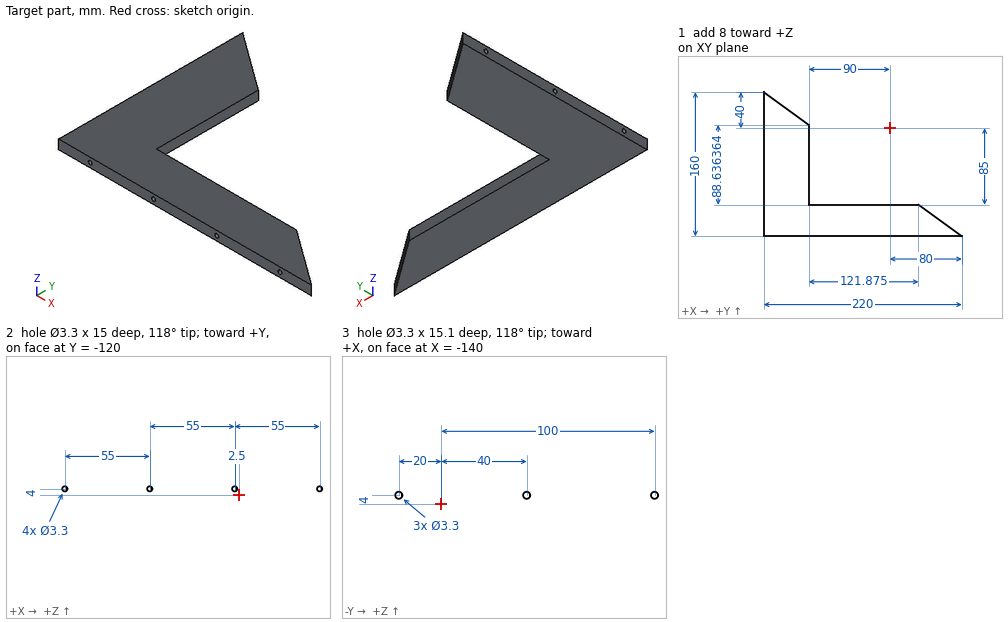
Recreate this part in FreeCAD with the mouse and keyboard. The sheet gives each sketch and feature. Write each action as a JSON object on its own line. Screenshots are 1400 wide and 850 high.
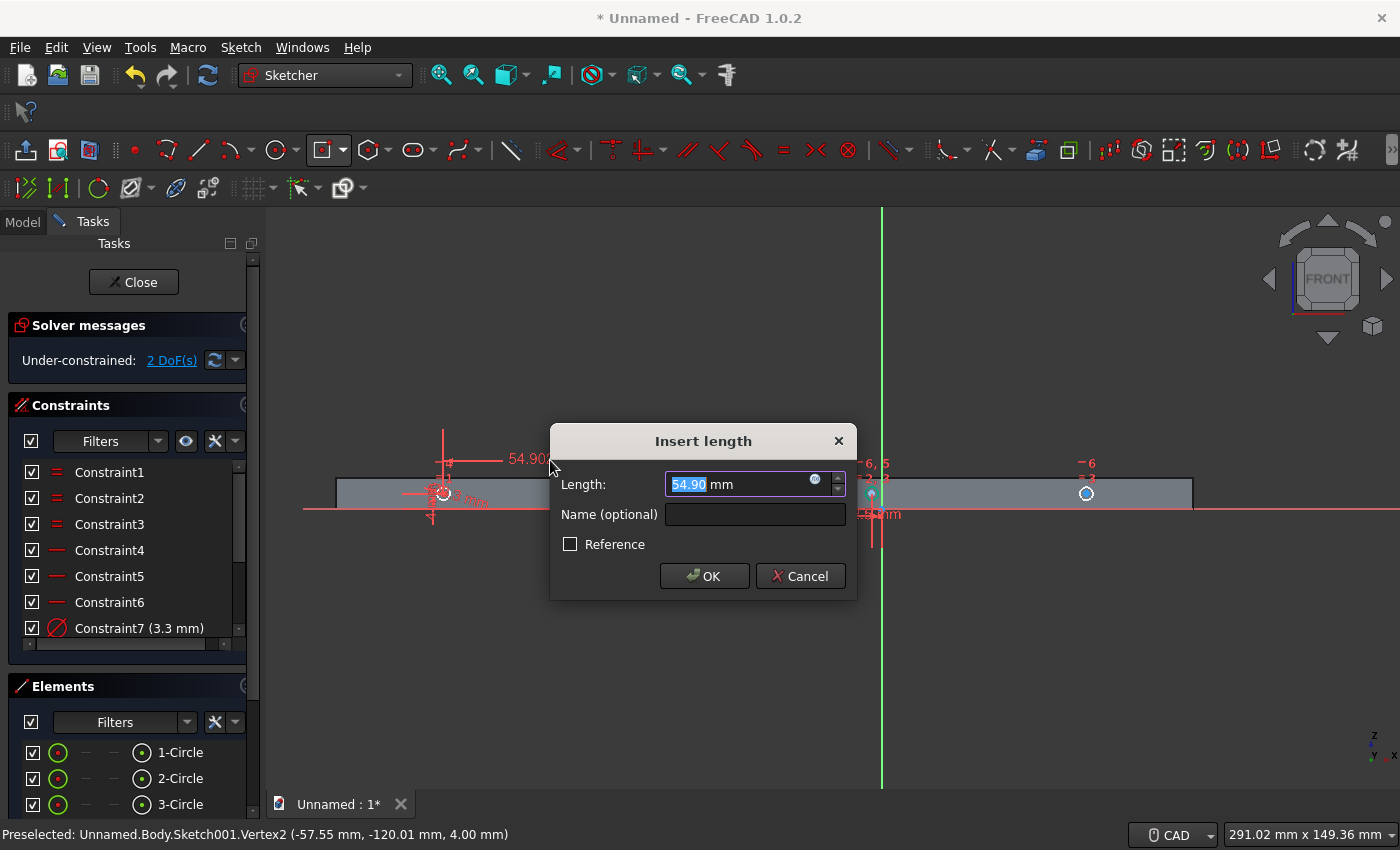
{"action": "type", "text": "55"}
{"action": "key", "text": "Return"}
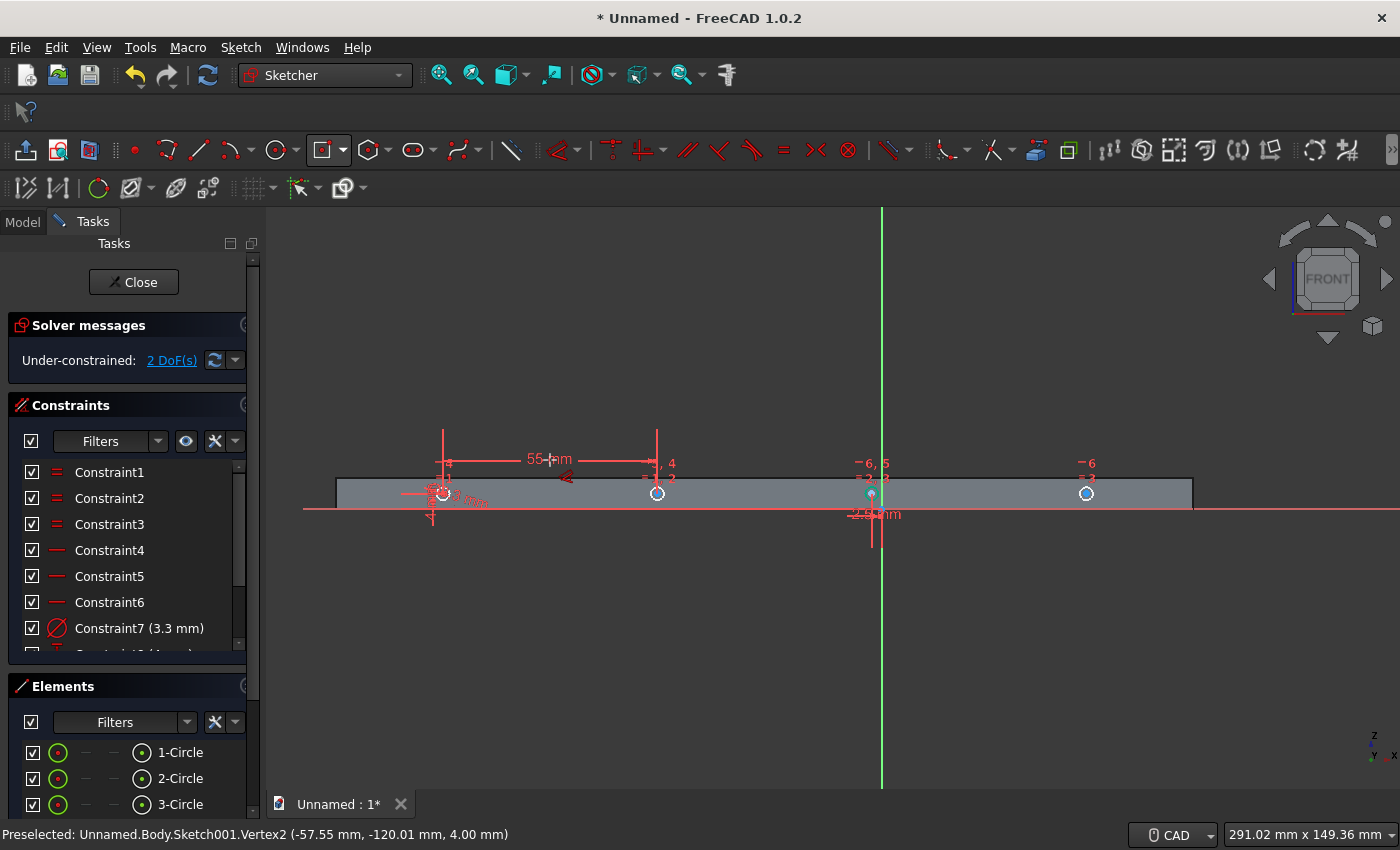
{"action": "left_click", "coordinate": [657, 494]}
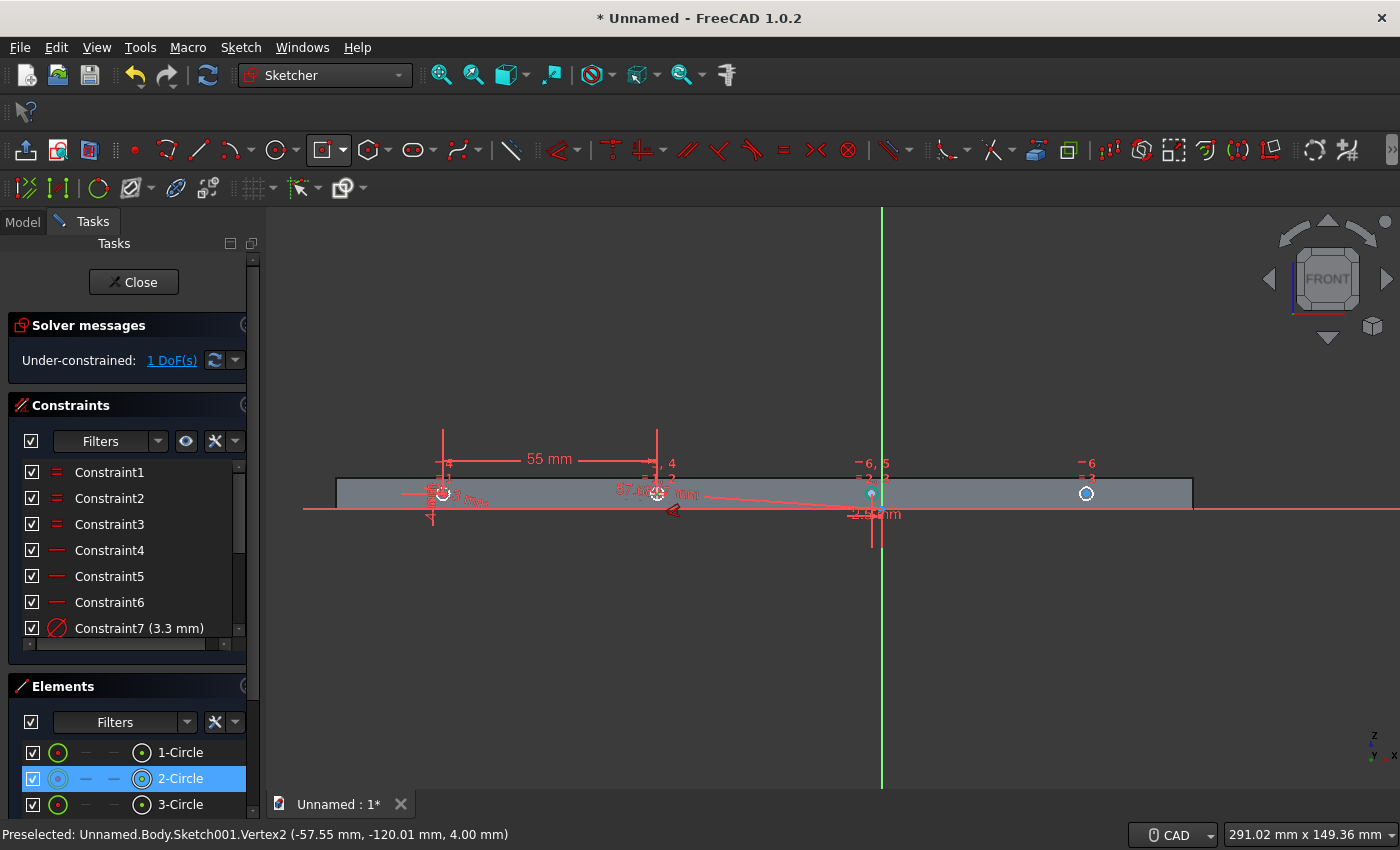
{"action": "left_click", "coordinate": [872, 494]}
{"action": "left_click", "coordinate": [765, 460]}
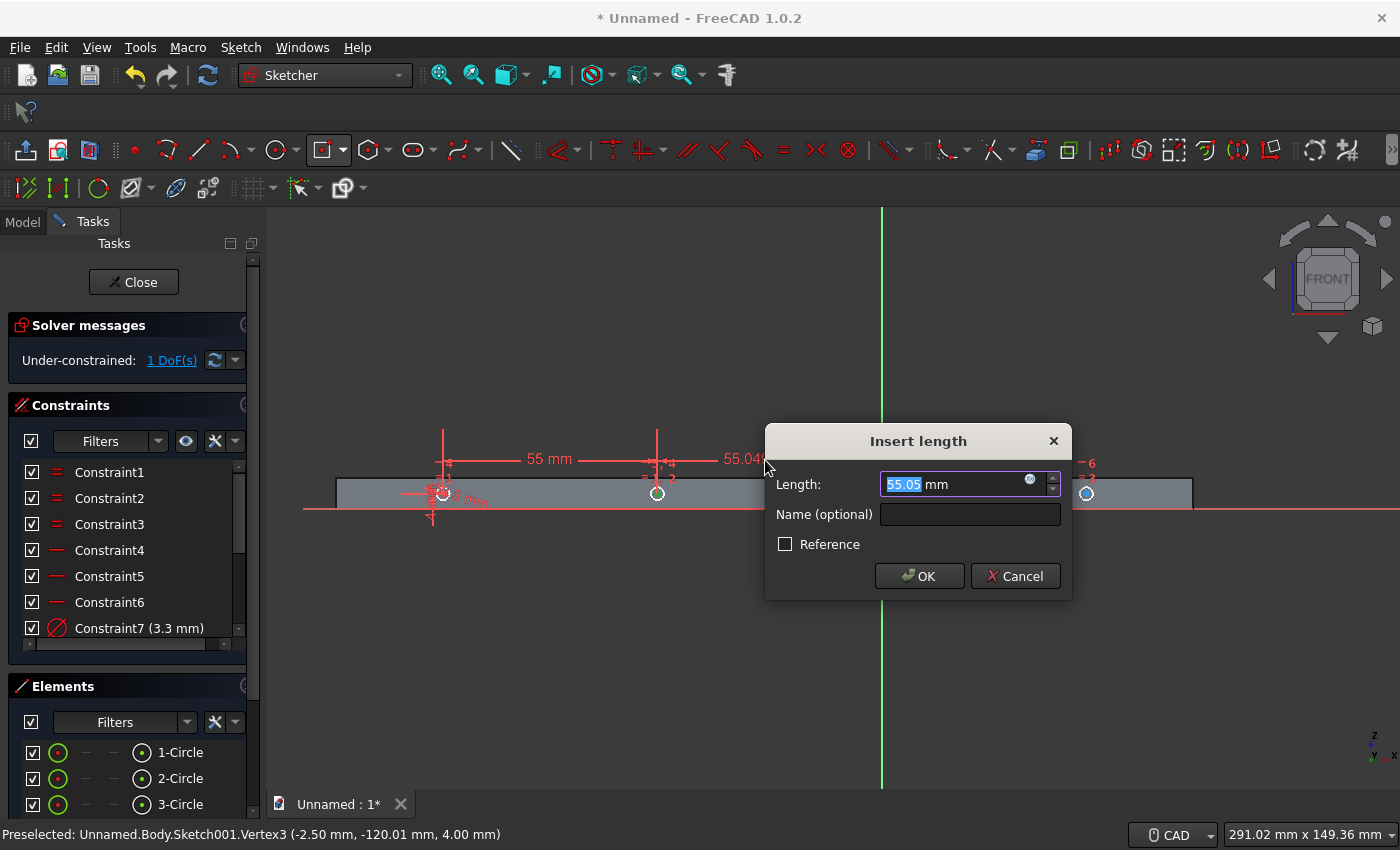
{"action": "type", "text": "55"}
{"action": "key", "text": "Return"}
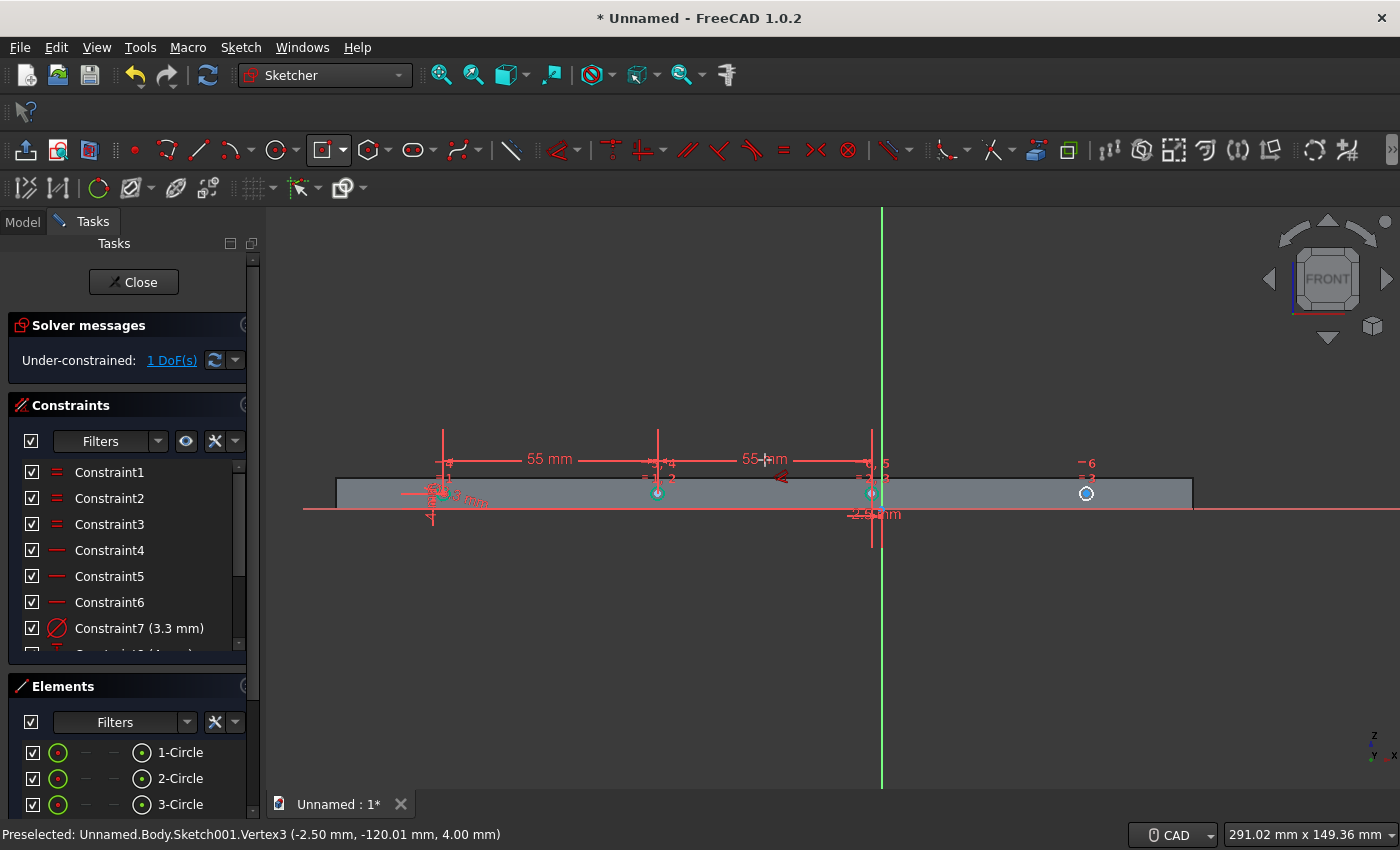
{"action": "left_click", "coordinate": [872, 494]}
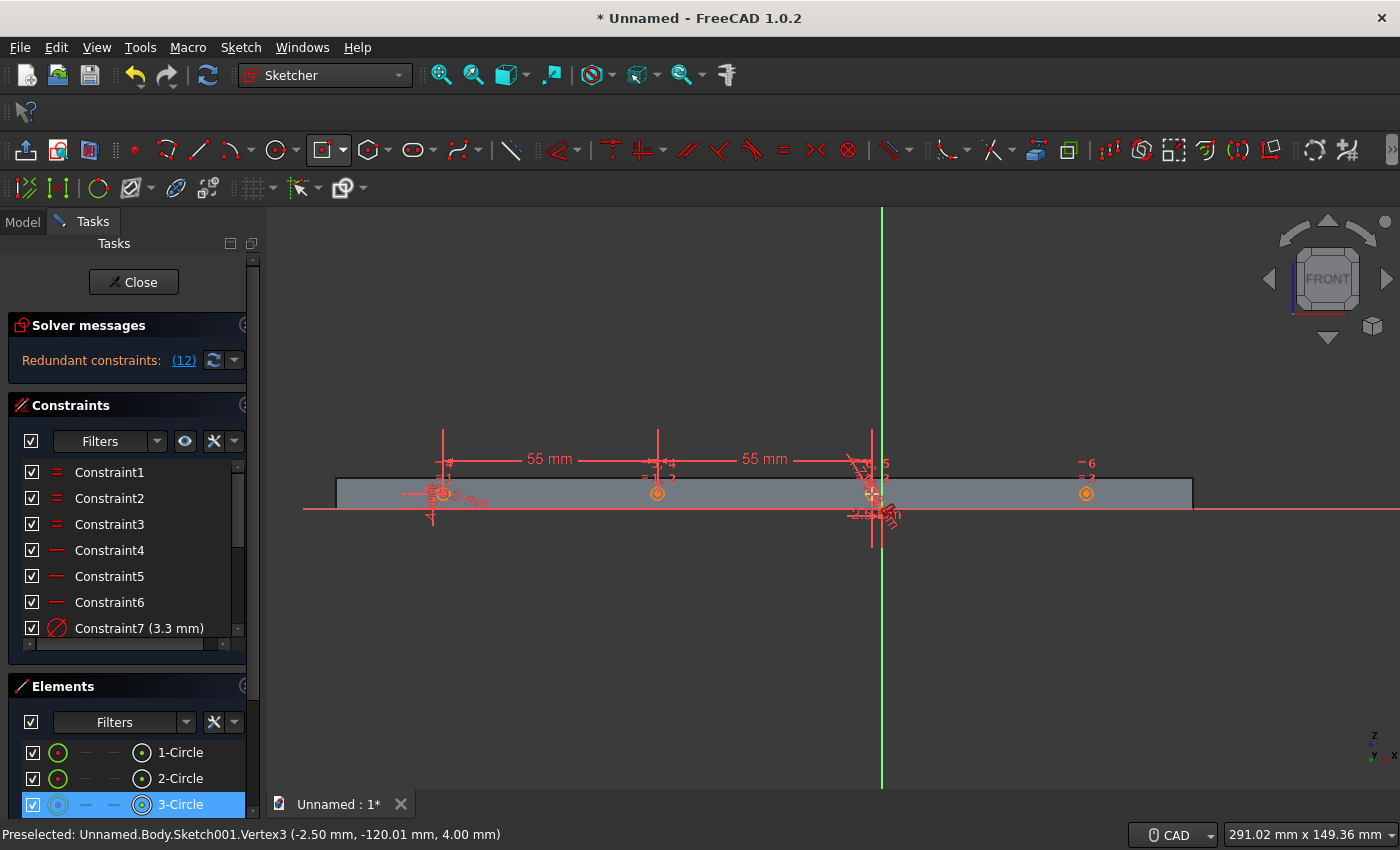
{"action": "left_click", "coordinate": [1086, 494]}
{"action": "left_click", "coordinate": [979, 460]}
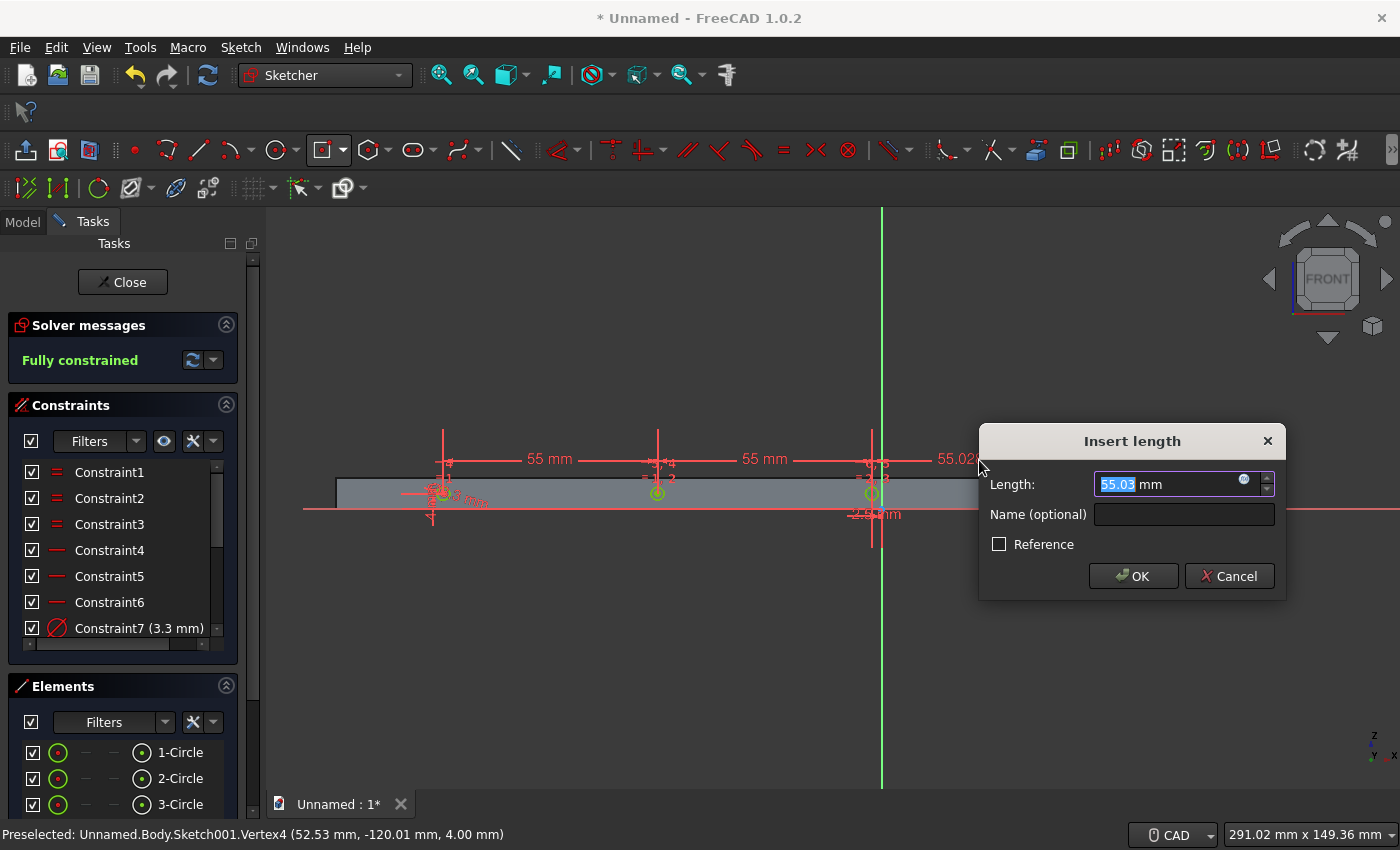
{"action": "type", "text": "55"}
{"action": "key", "text": "Return"}
{"action": "key", "text": "Escape"}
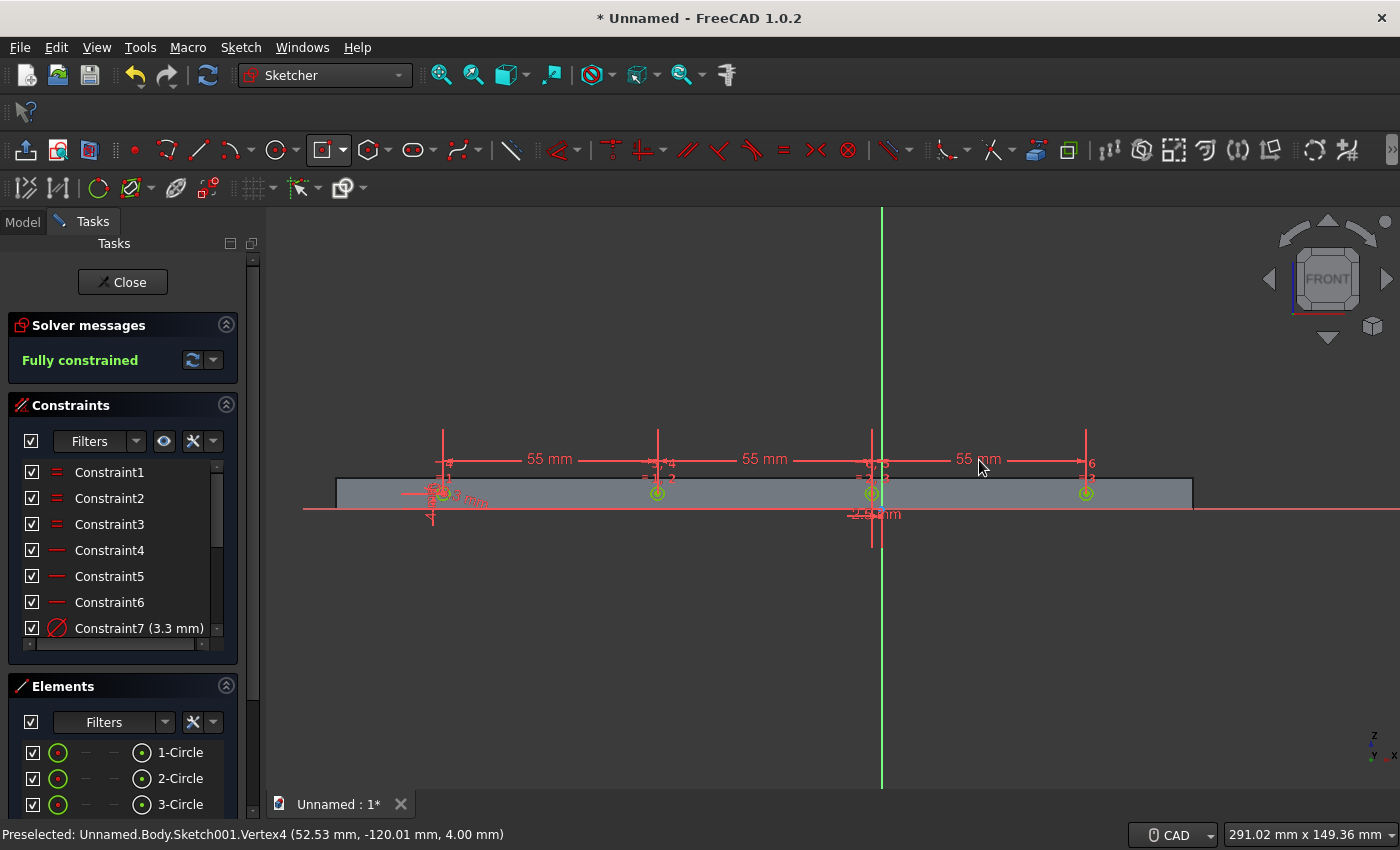
{"action": "left_click", "coordinate": [123, 282]}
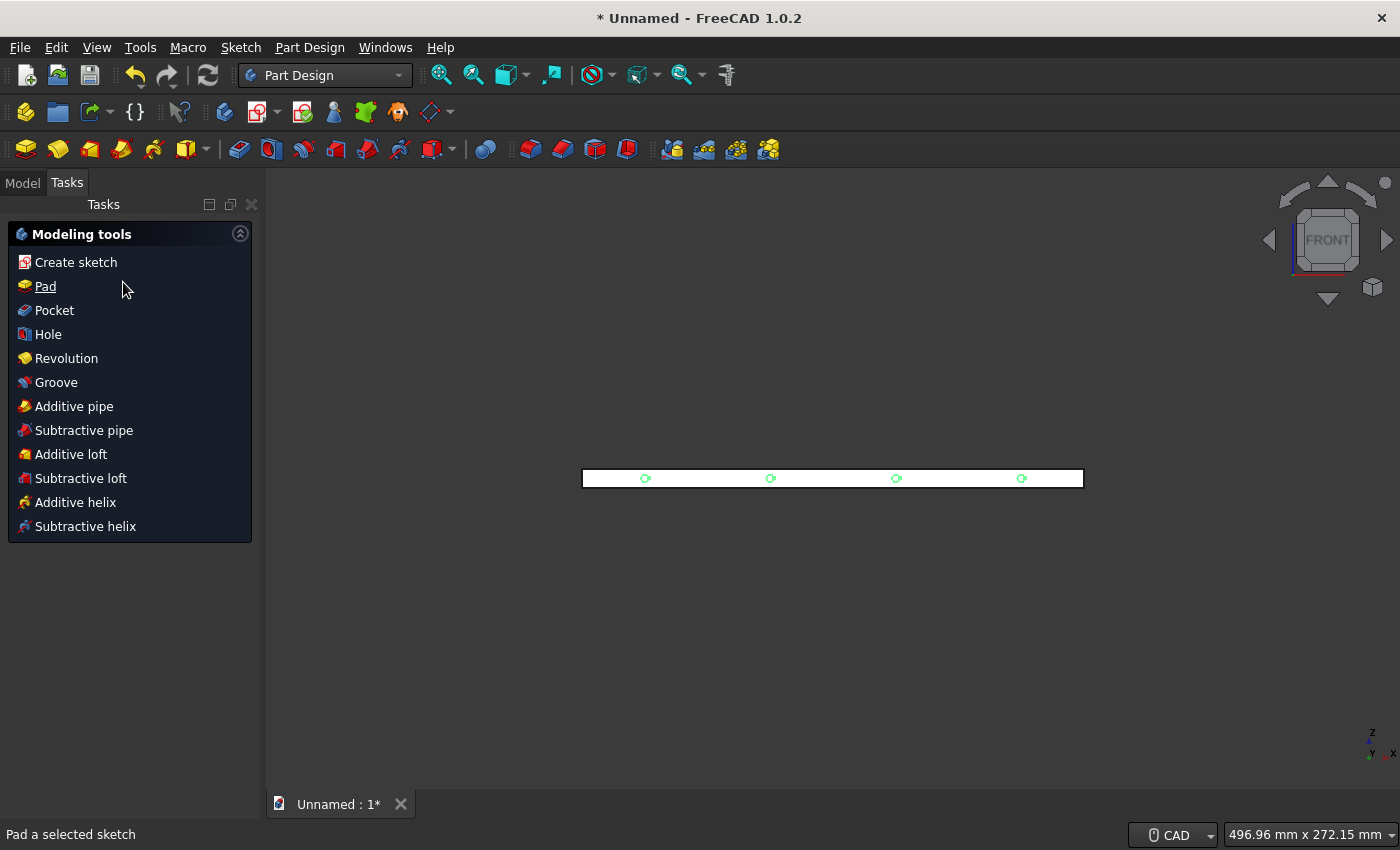
{"action": "left_click", "coordinate": [272, 150]}